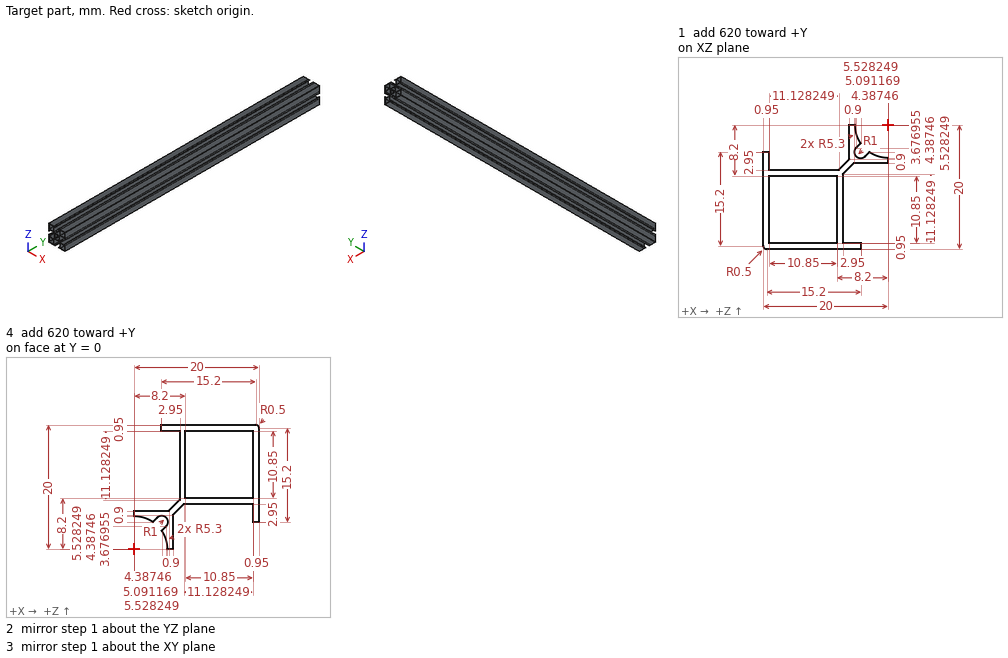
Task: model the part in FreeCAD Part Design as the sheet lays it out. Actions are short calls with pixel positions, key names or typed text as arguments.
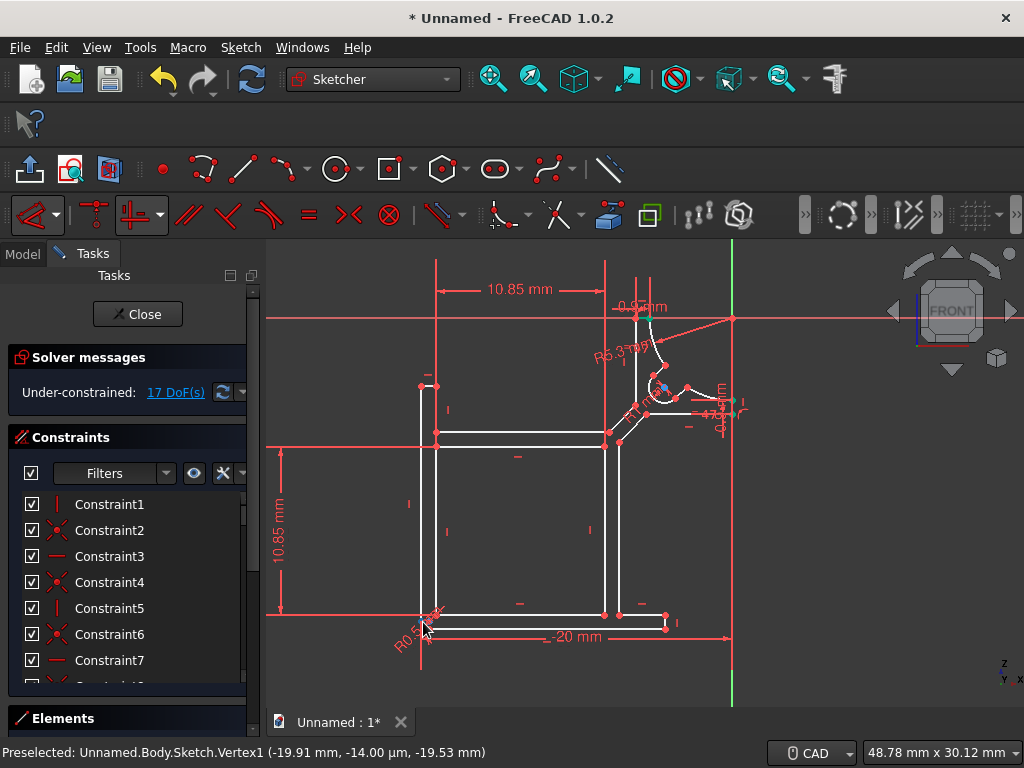
click(665, 629)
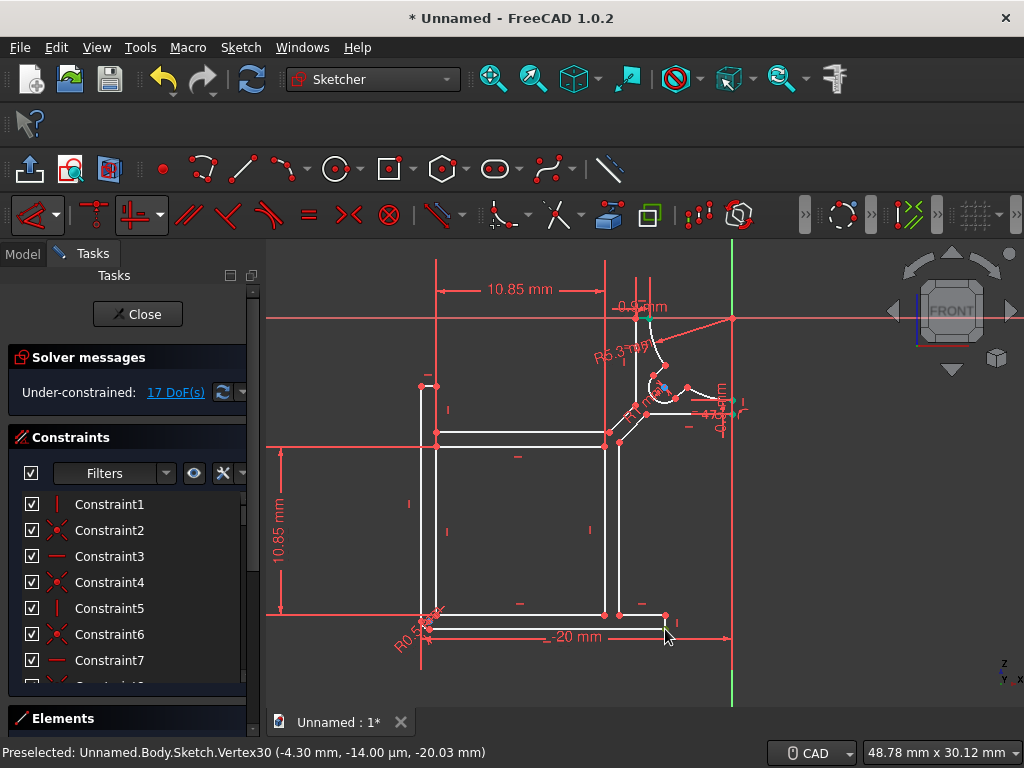
click(58, 216)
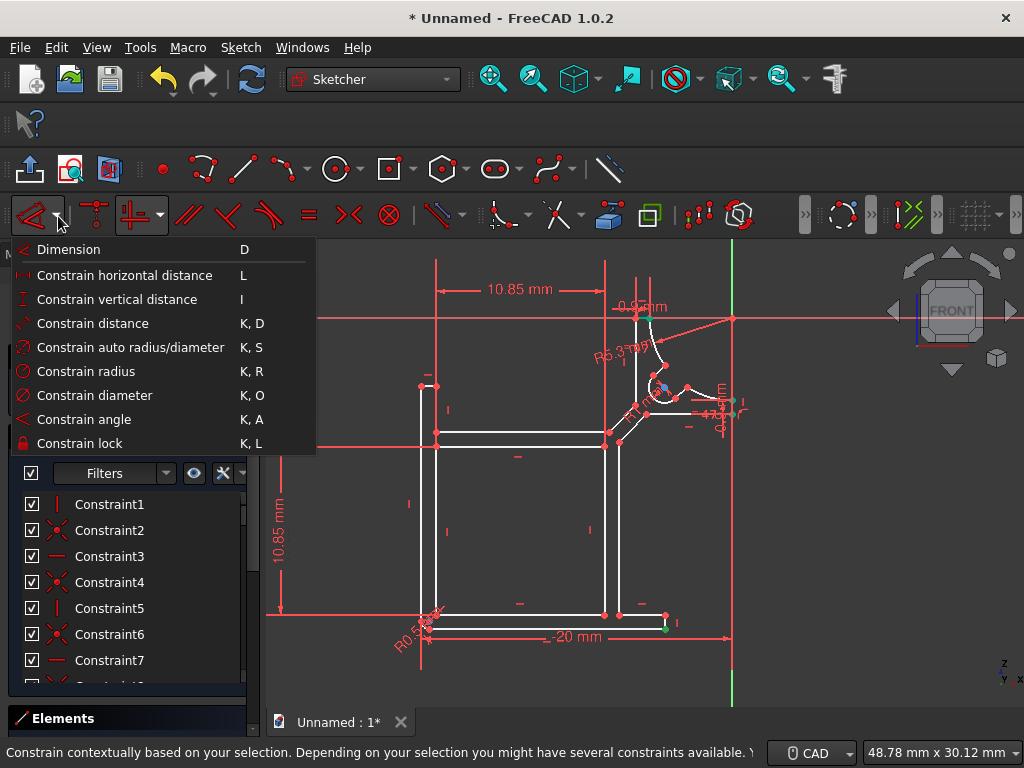
click(164, 299)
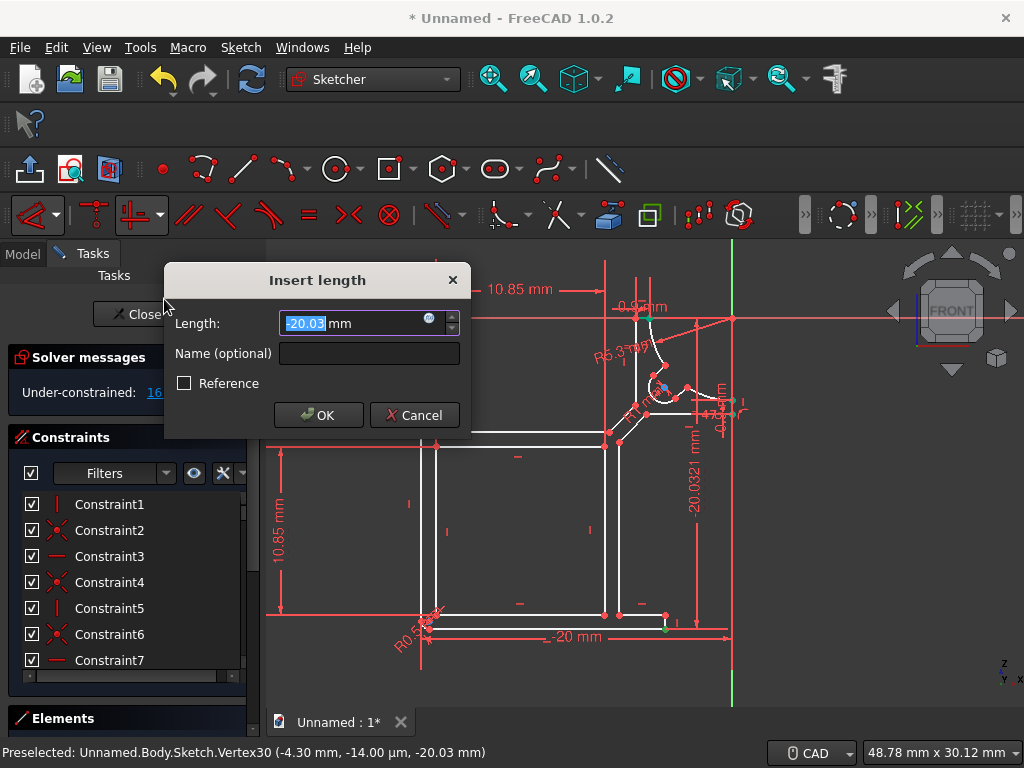
text(-20)
key(Return)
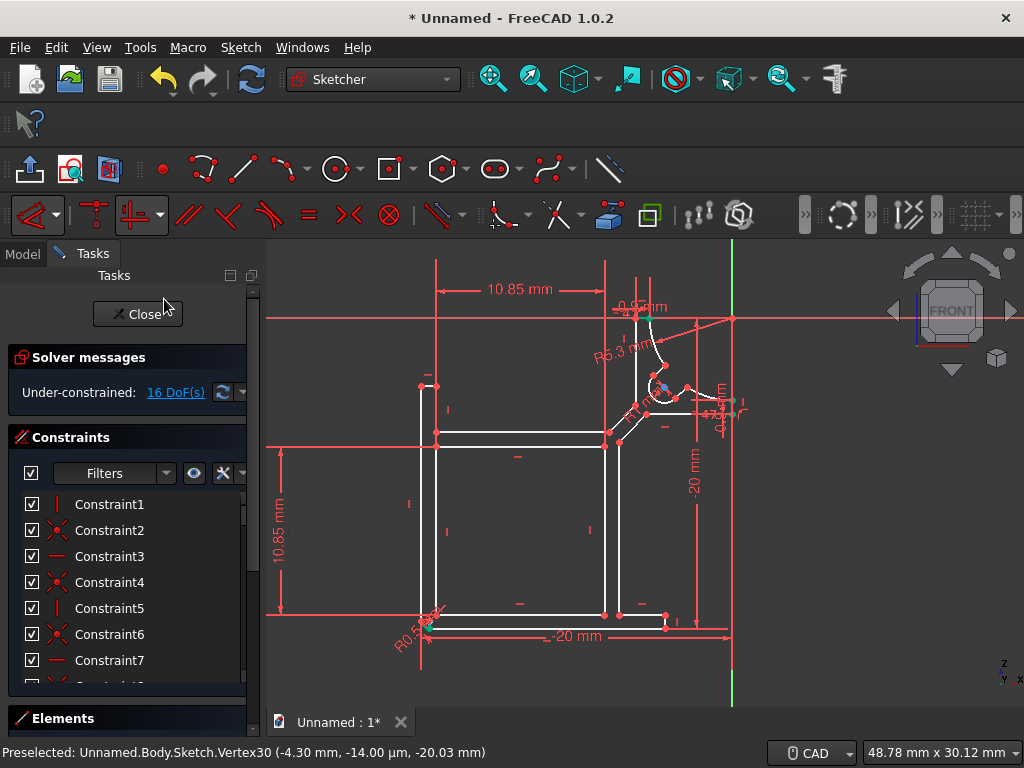
click(421, 551)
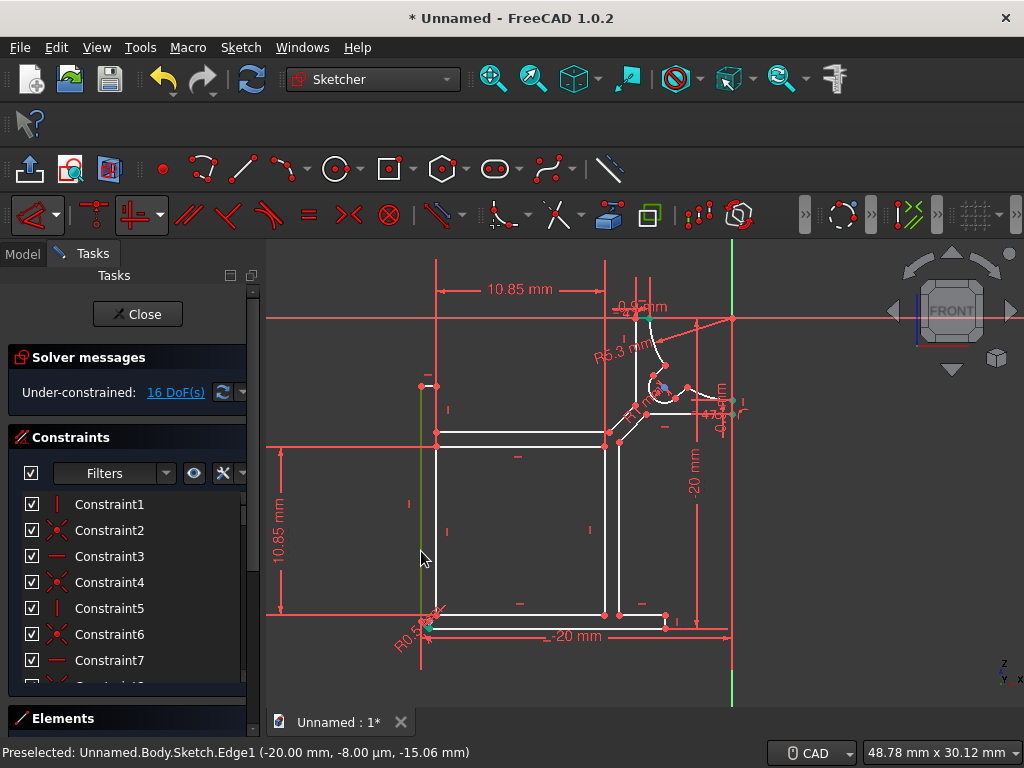
click(58, 216)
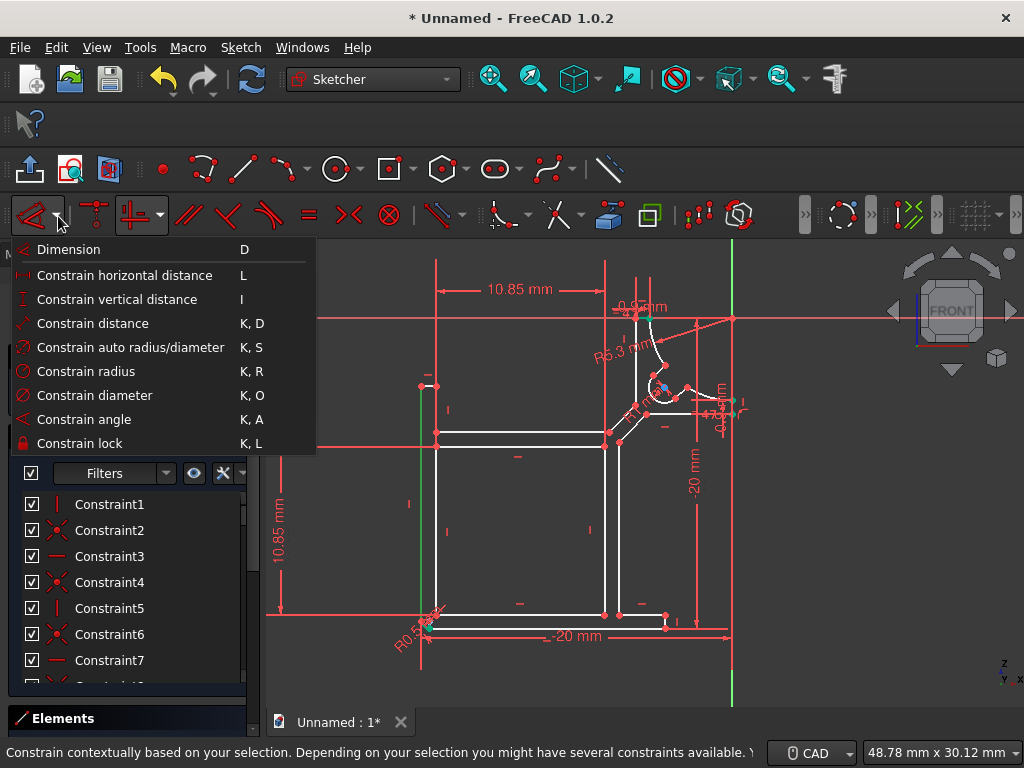
click(164, 299)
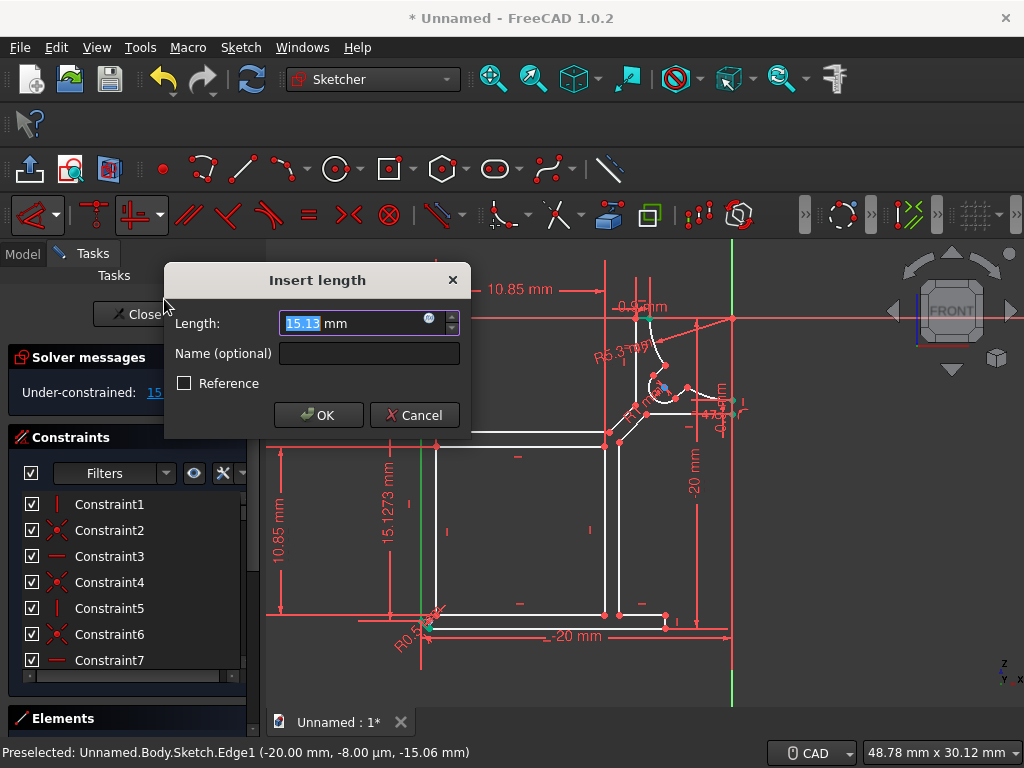
text(15.2)
key(Return)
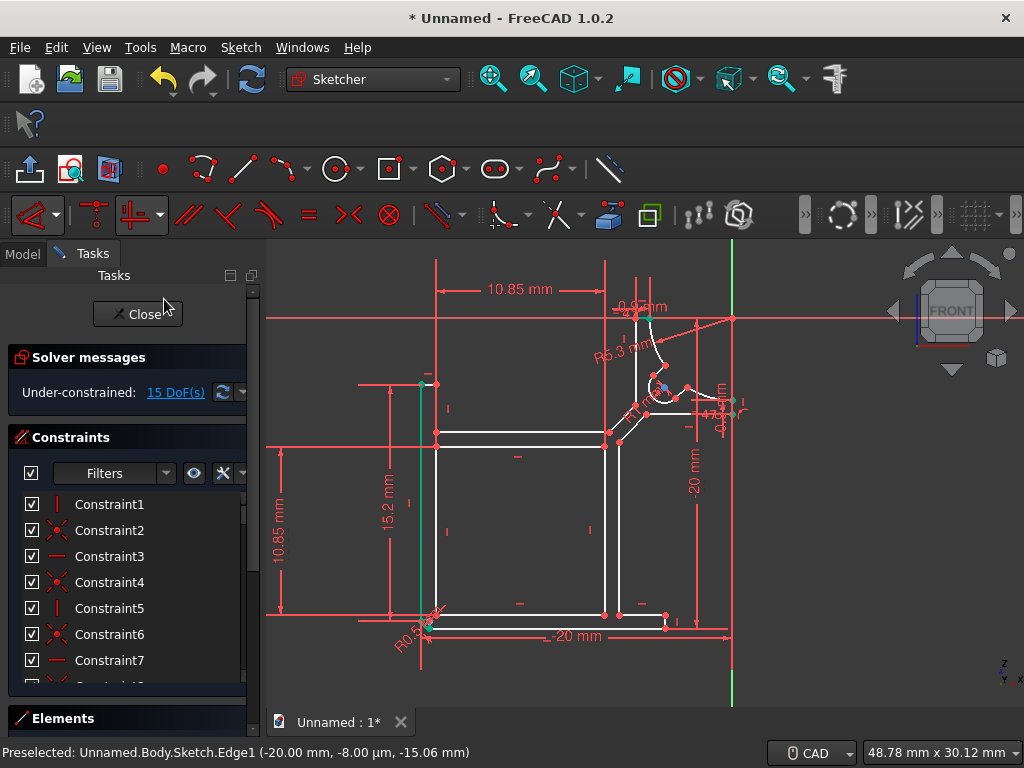
scroll(429, 385, up, 5)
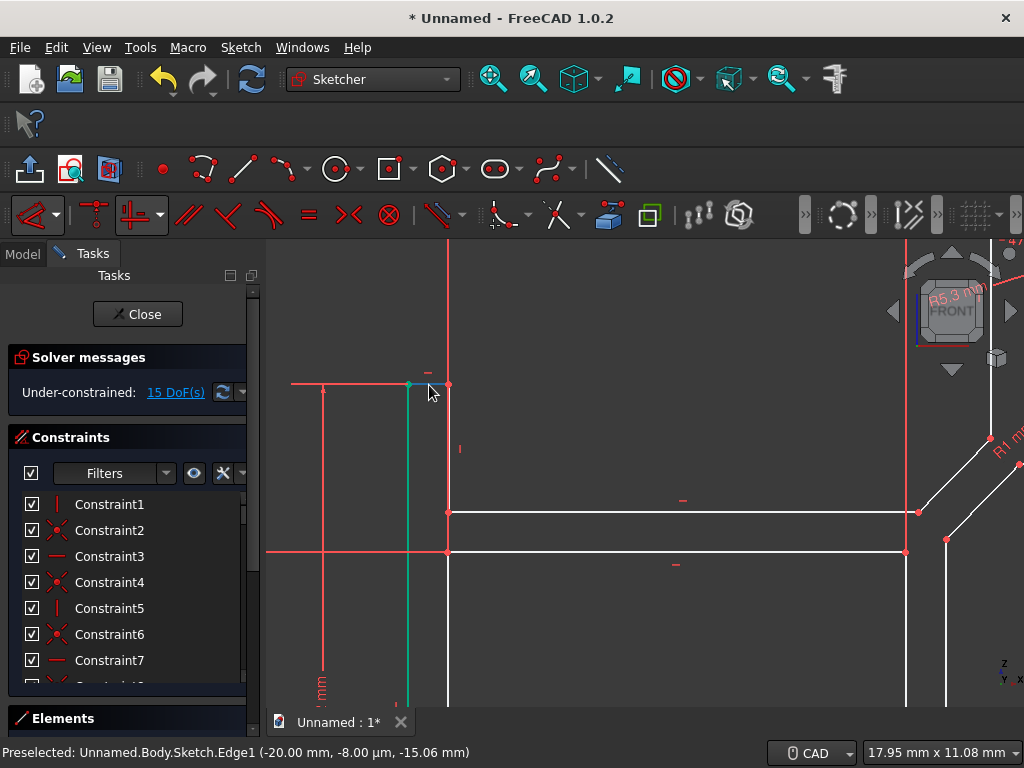
click(428, 384)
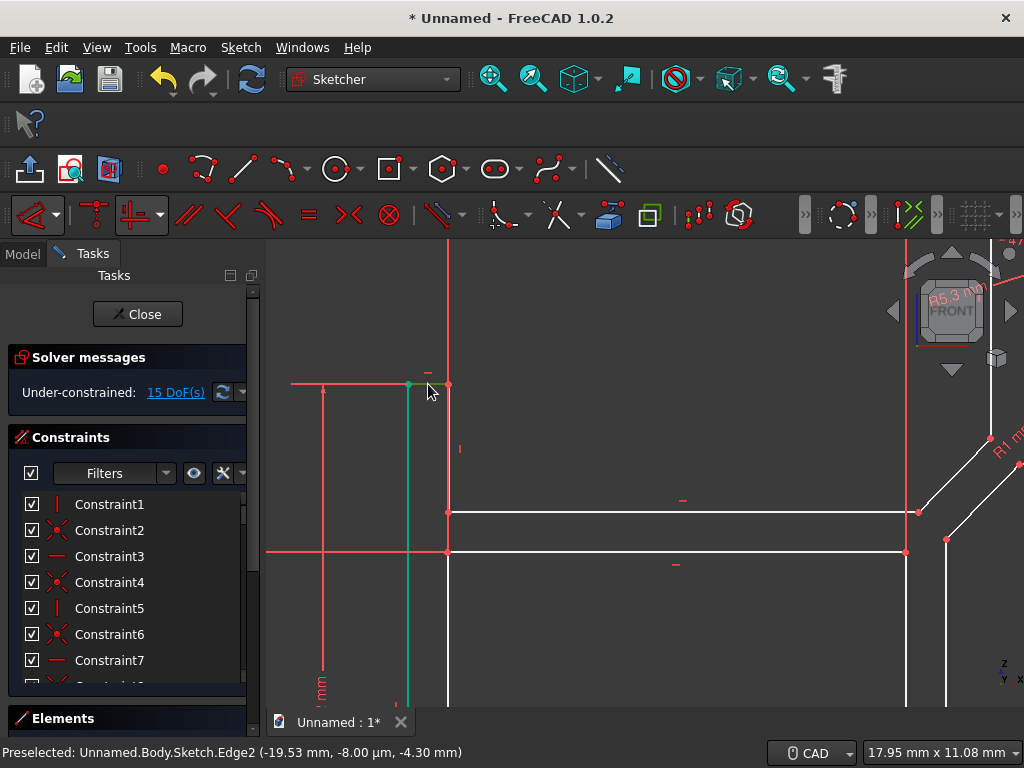
click(58, 216)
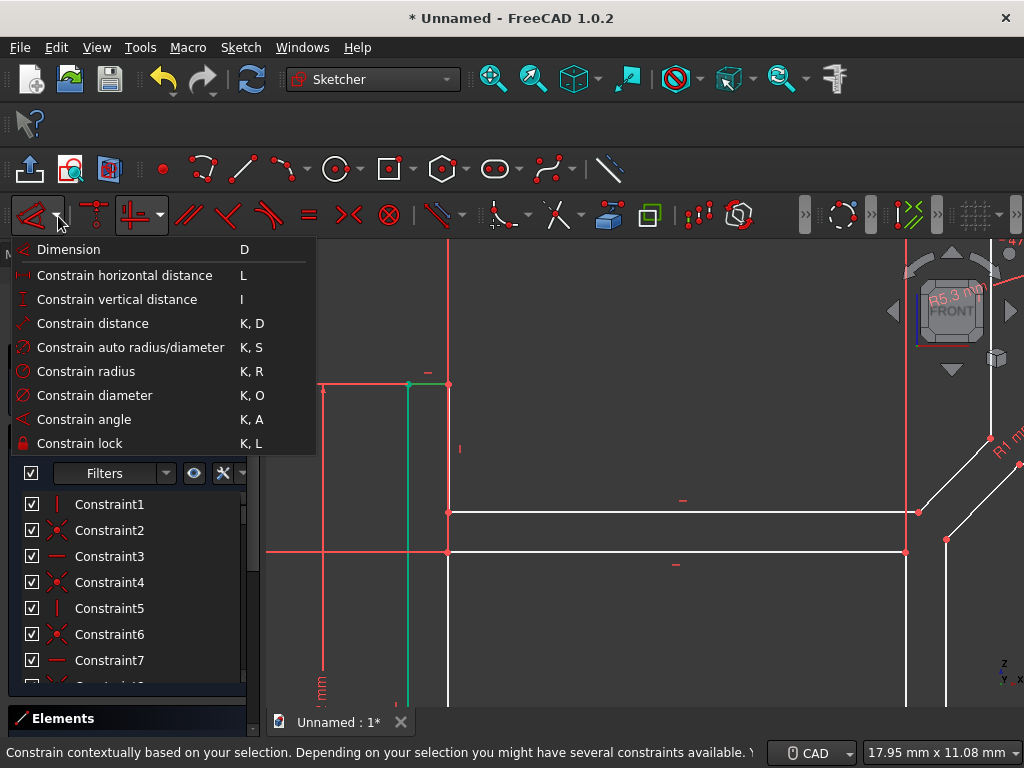
click(164, 275)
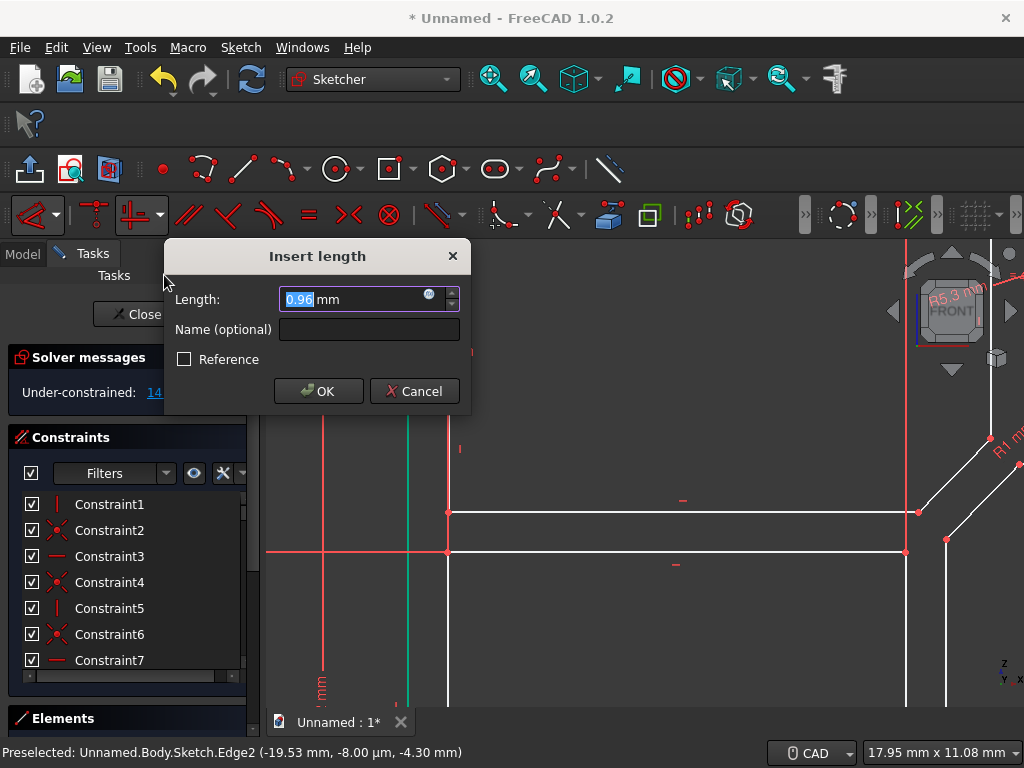
text(0.95)
key(Return)